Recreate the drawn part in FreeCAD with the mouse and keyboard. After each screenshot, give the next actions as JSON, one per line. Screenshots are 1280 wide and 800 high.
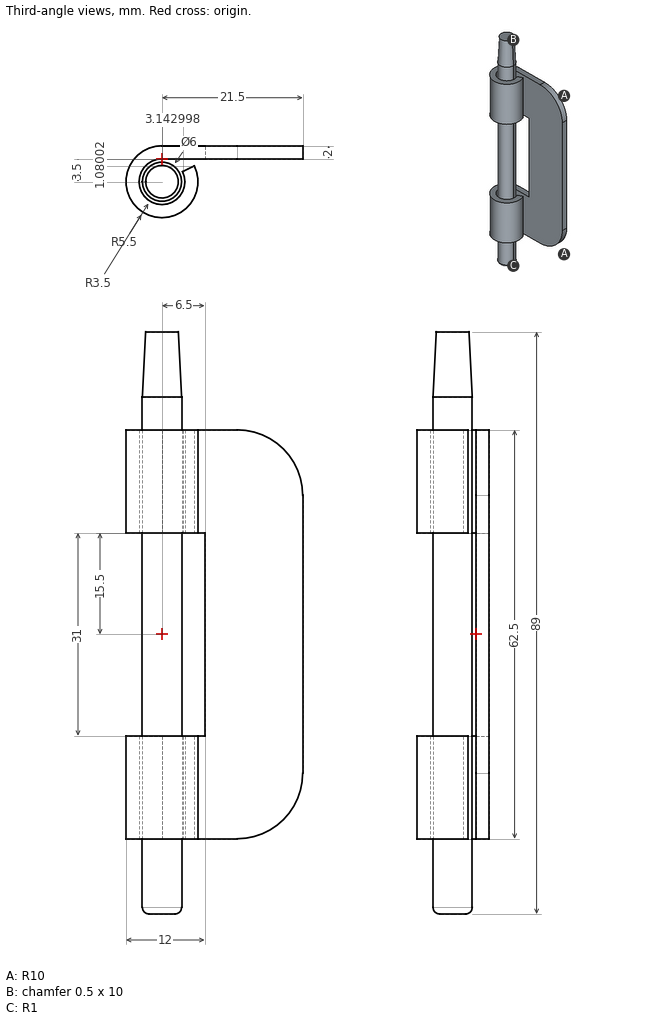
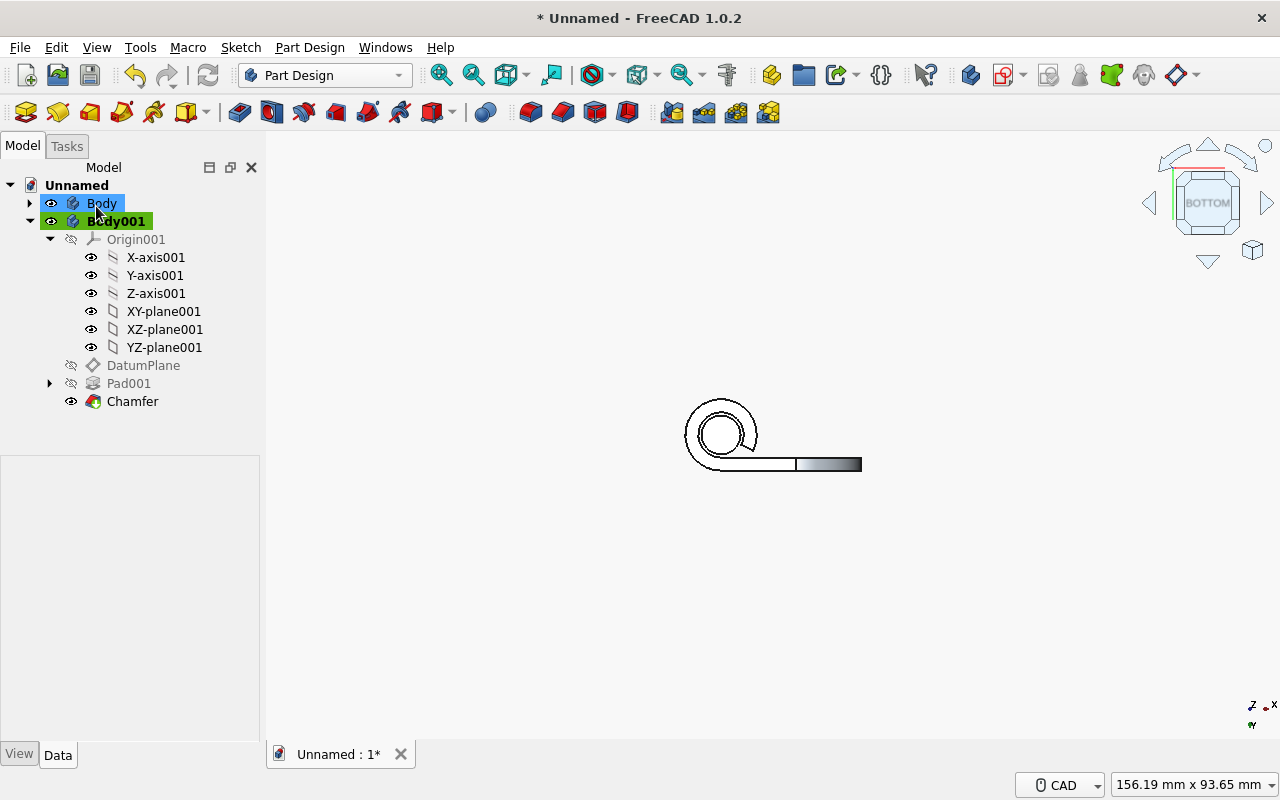
{"action": "key", "text": "v f"}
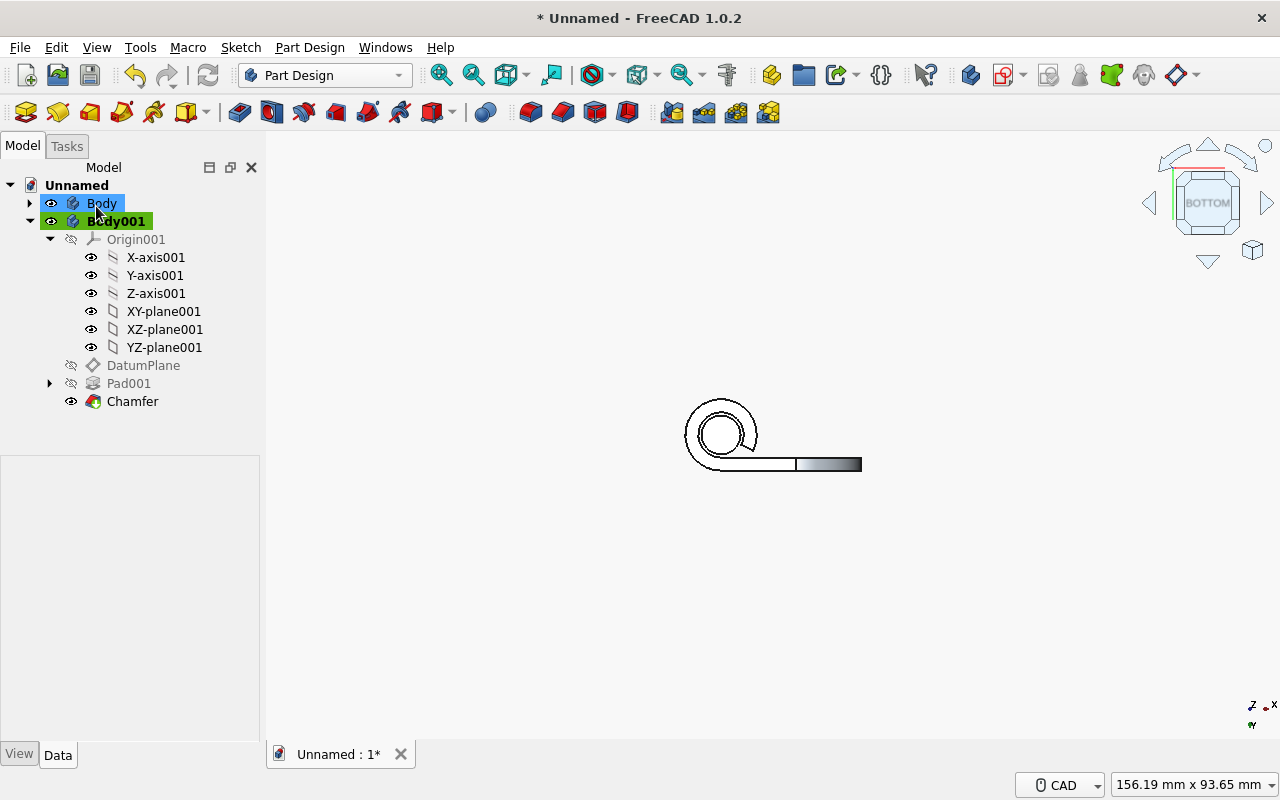
{"action": "left_click", "coordinate": [702, 434]}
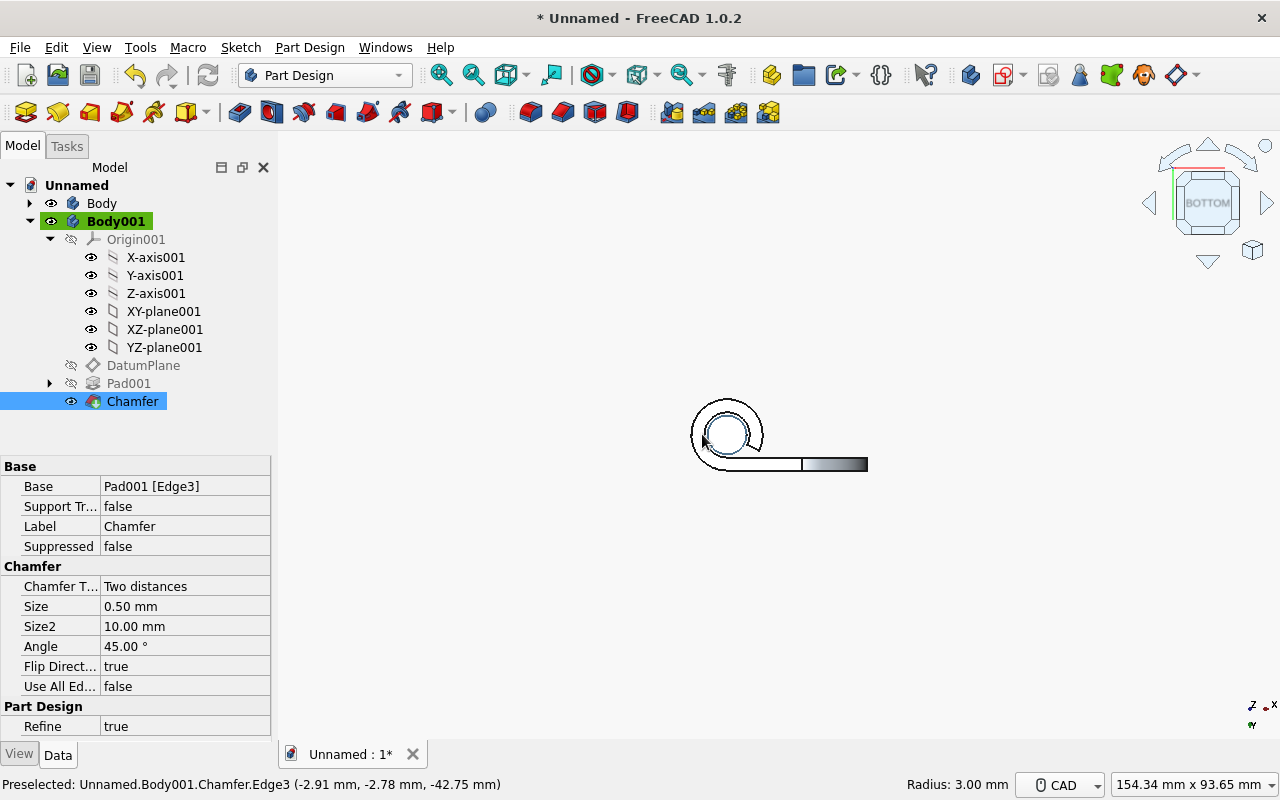
{"action": "left_click", "coordinate": [532, 112]}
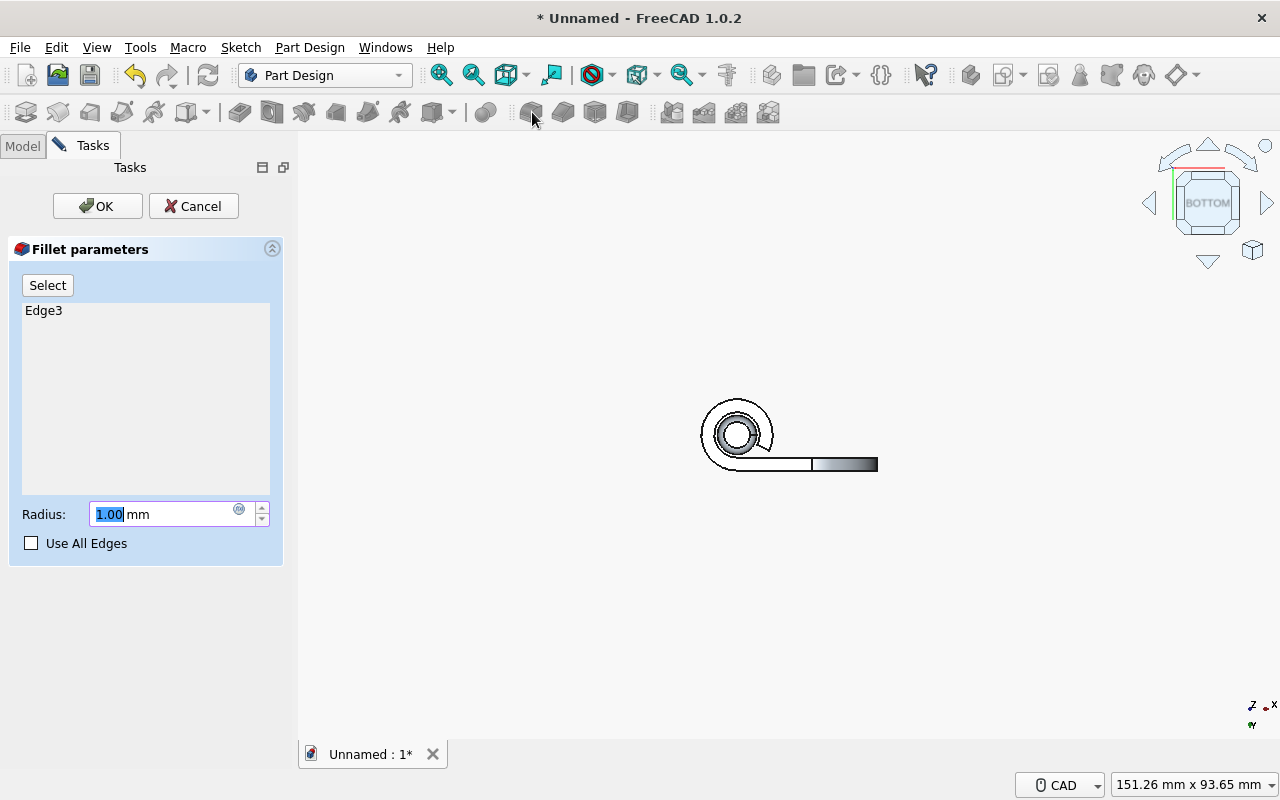
{"action": "type", "text": "1"}
{"action": "key", "text": "Tab"}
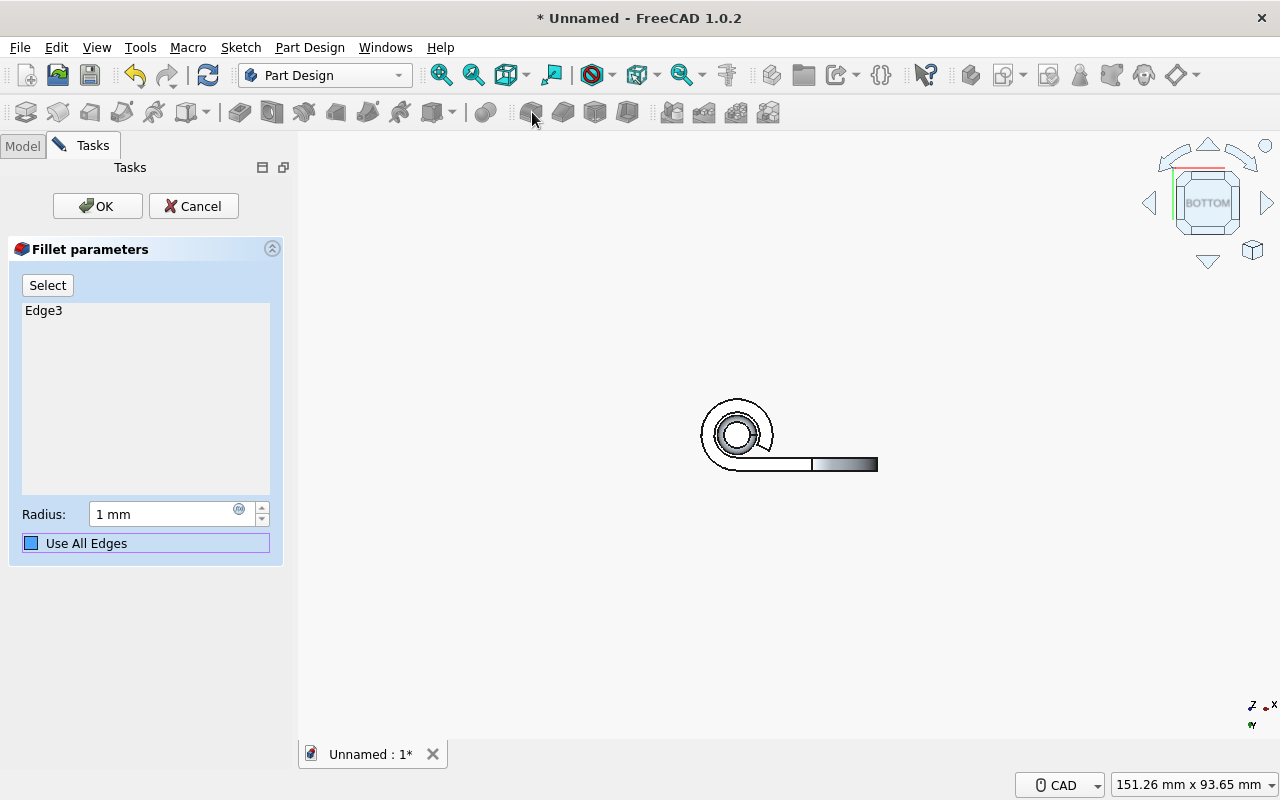
{"action": "left_click", "coordinate": [98, 206]}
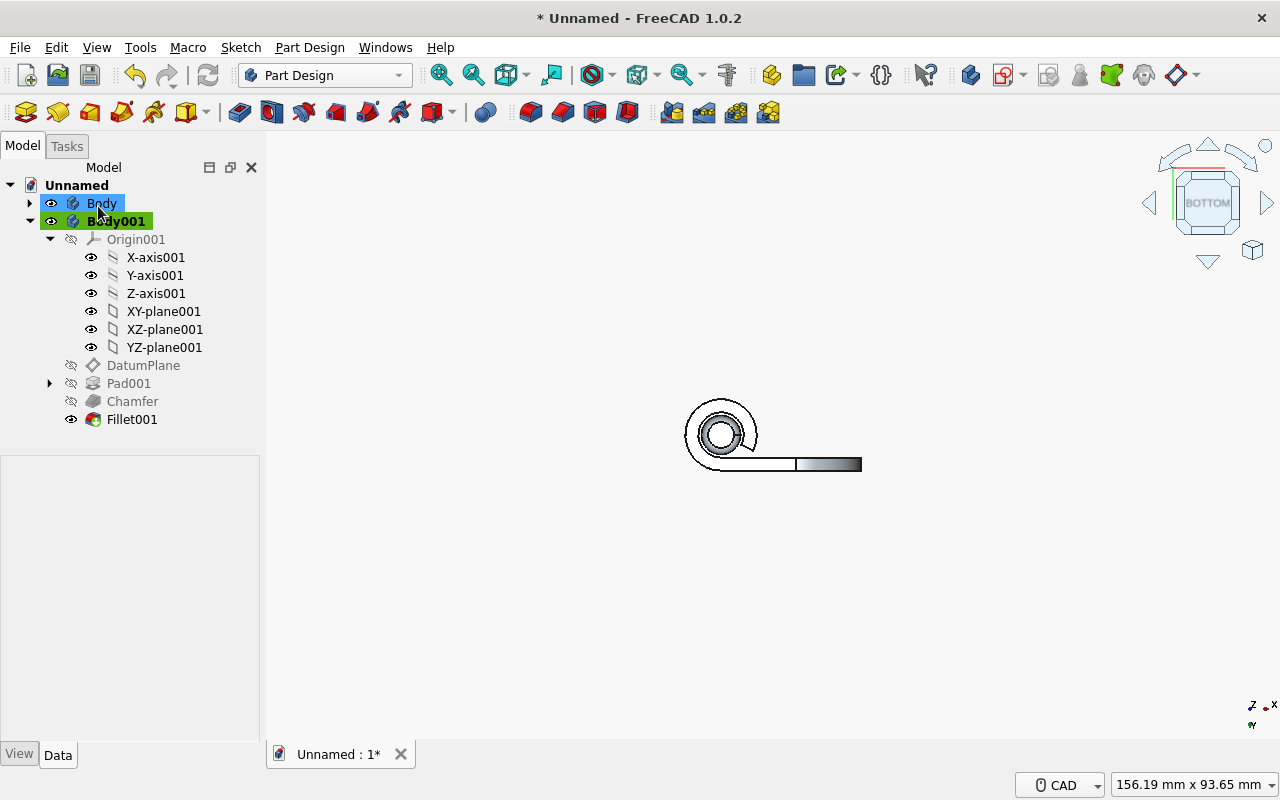
{"action": "key", "text": "0"}